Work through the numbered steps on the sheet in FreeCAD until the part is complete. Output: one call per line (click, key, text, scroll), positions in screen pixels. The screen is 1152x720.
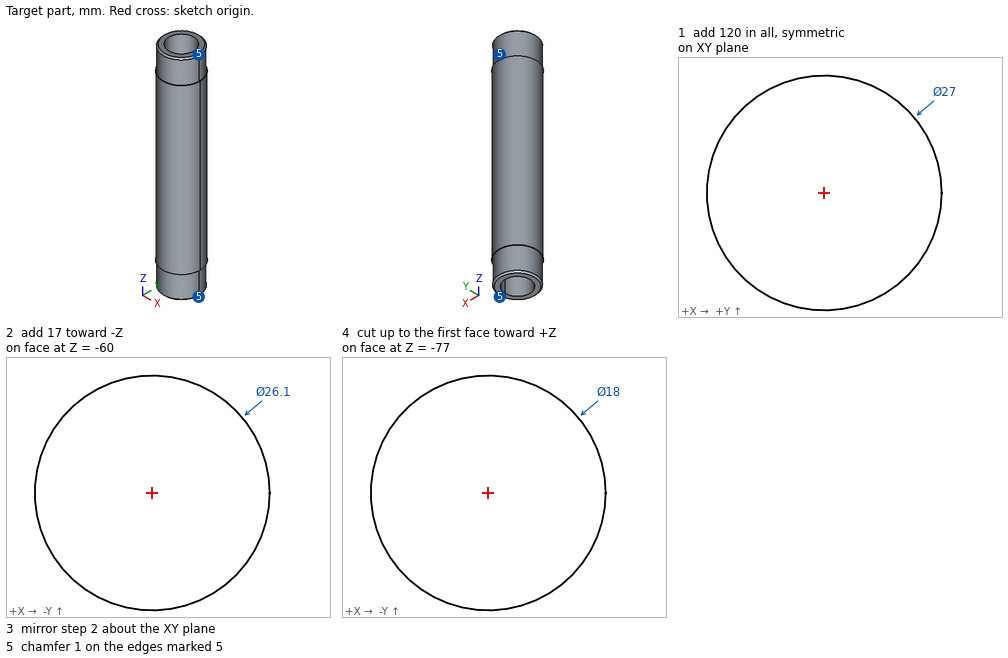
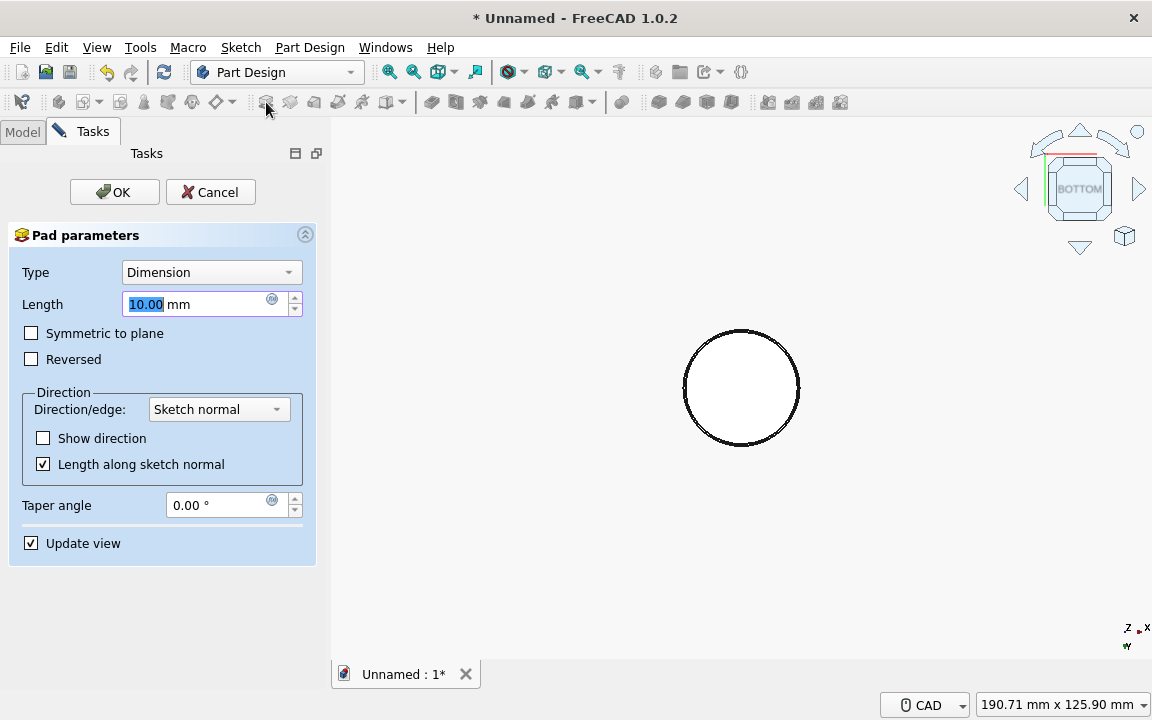
text(17)
key(Tab)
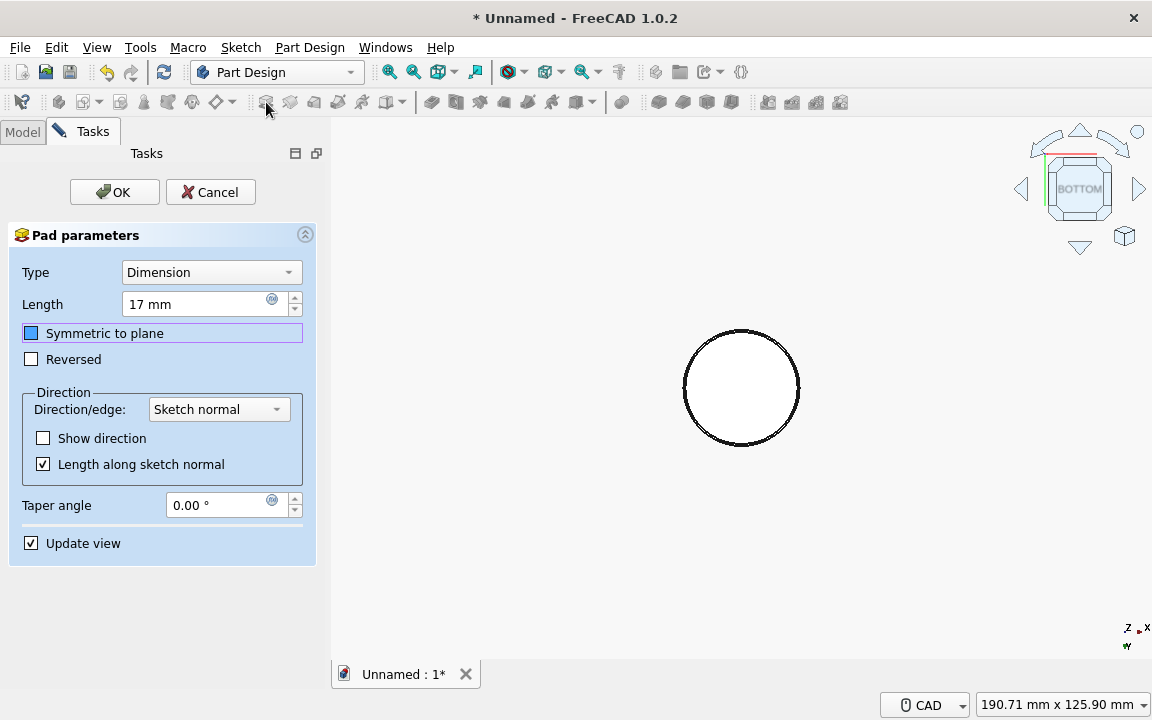
click(115, 192)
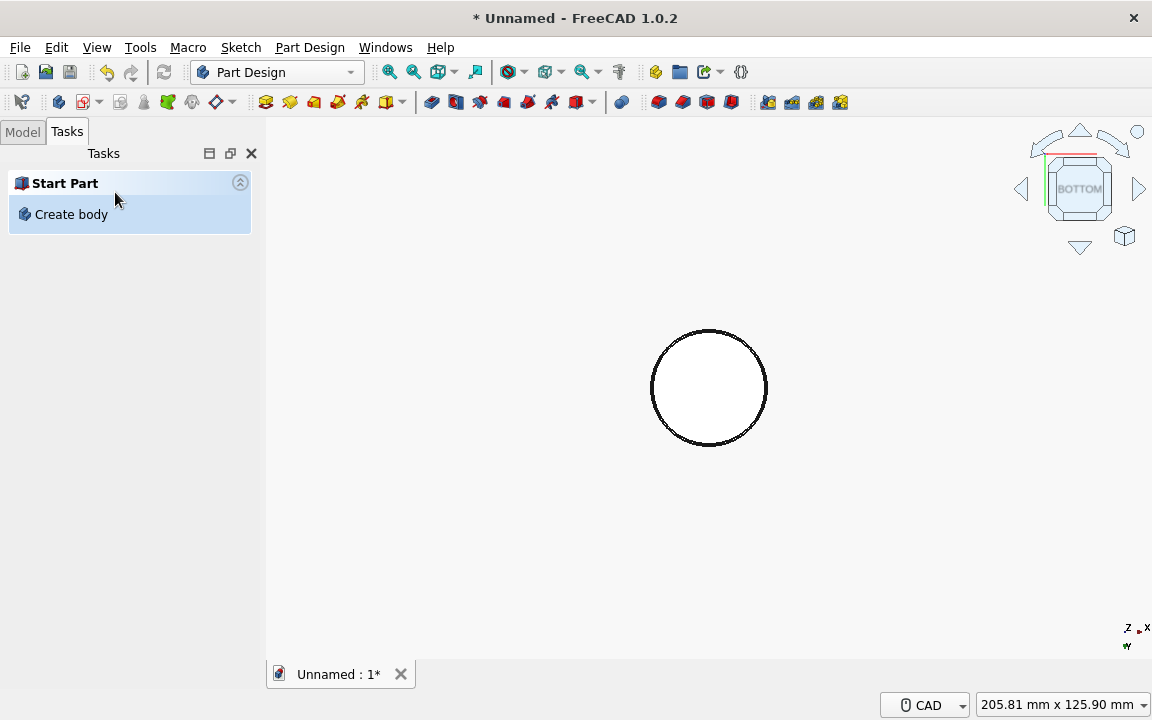
key(v)
key(f)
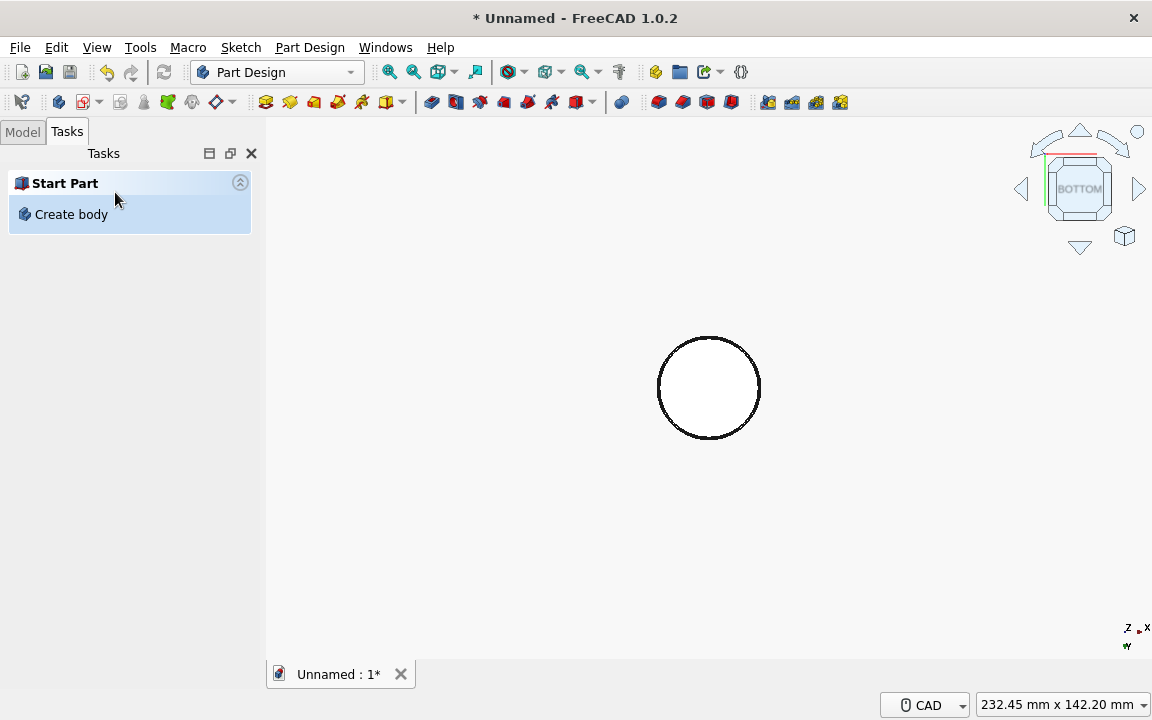
click(23, 131)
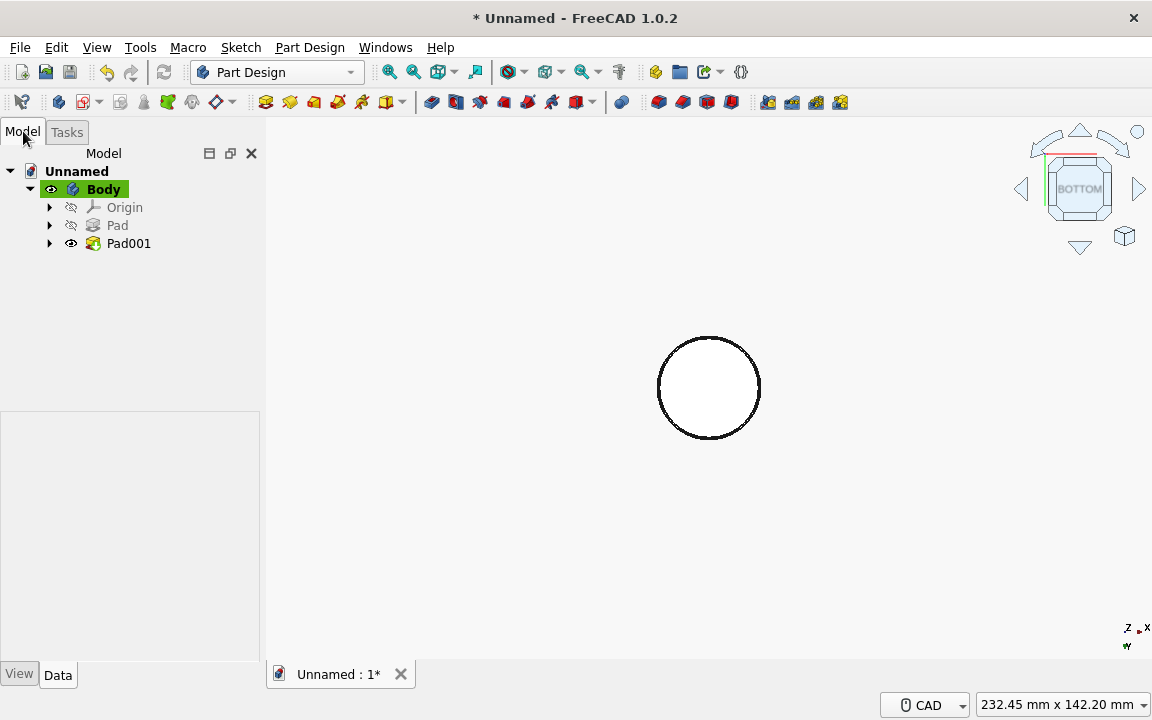
click(116, 243)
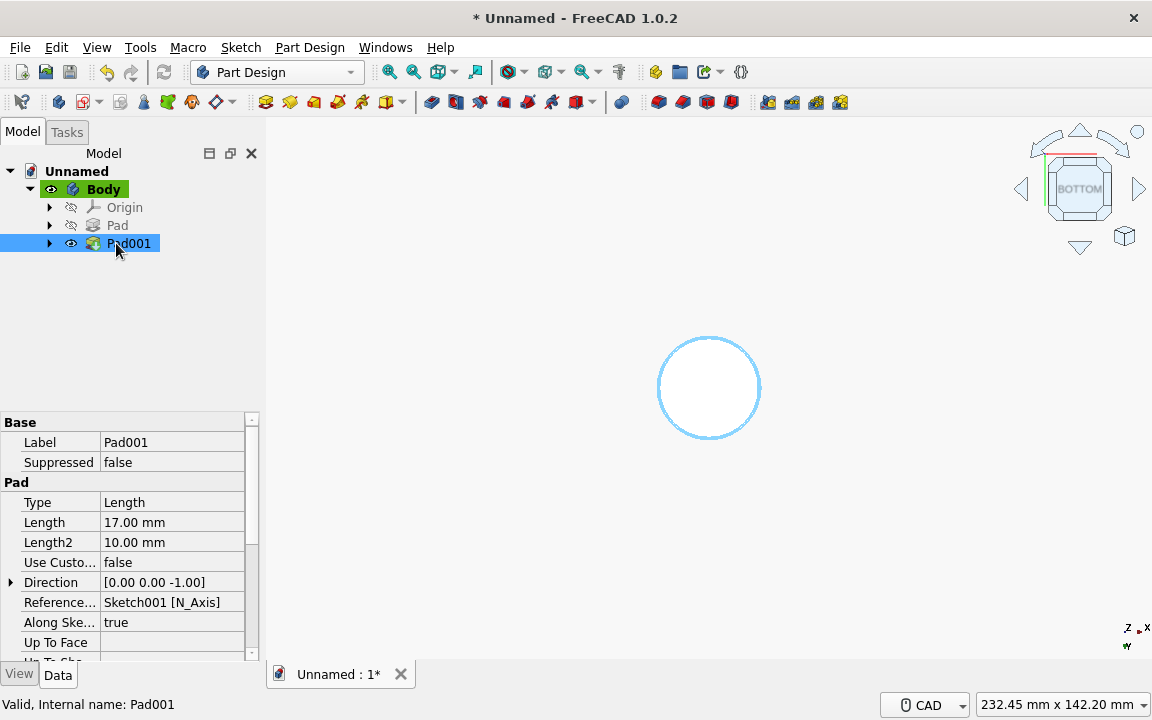
click(768, 102)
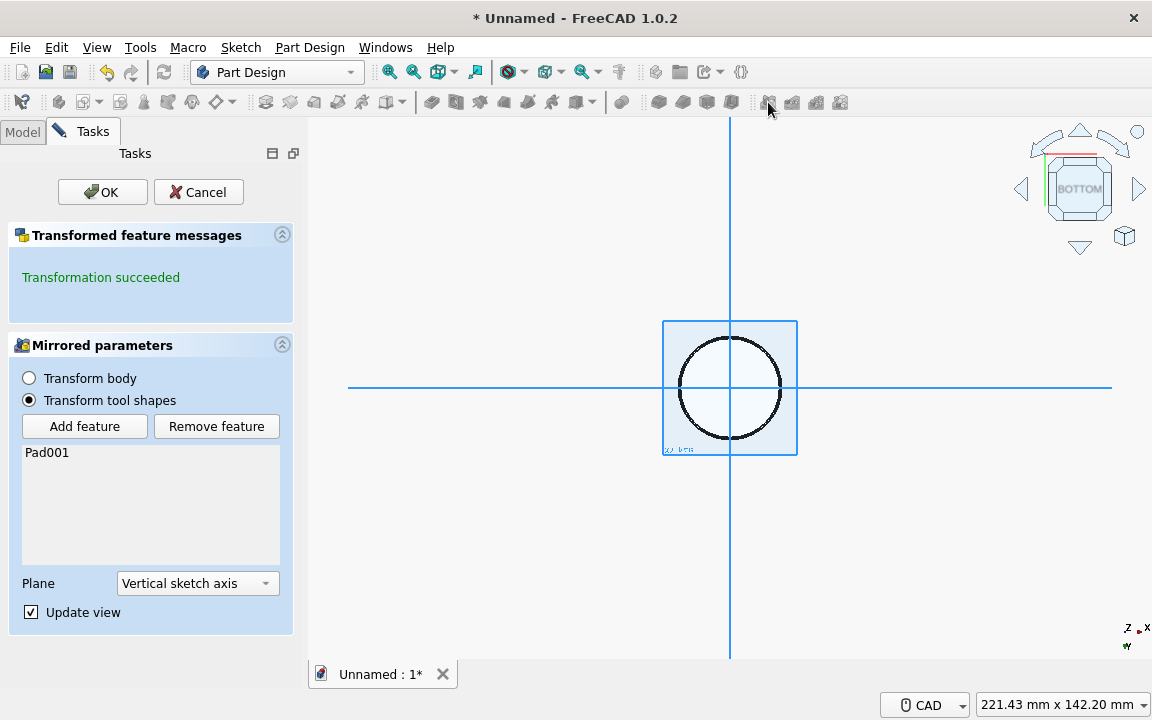
click(198, 584)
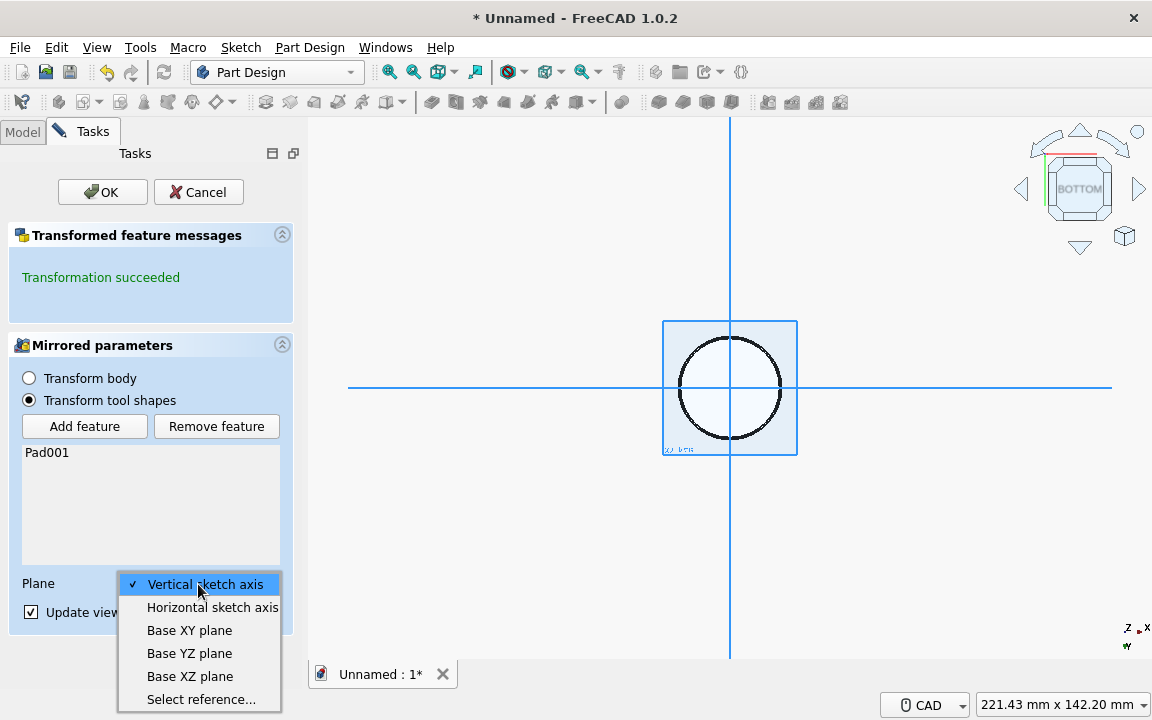
click(198, 630)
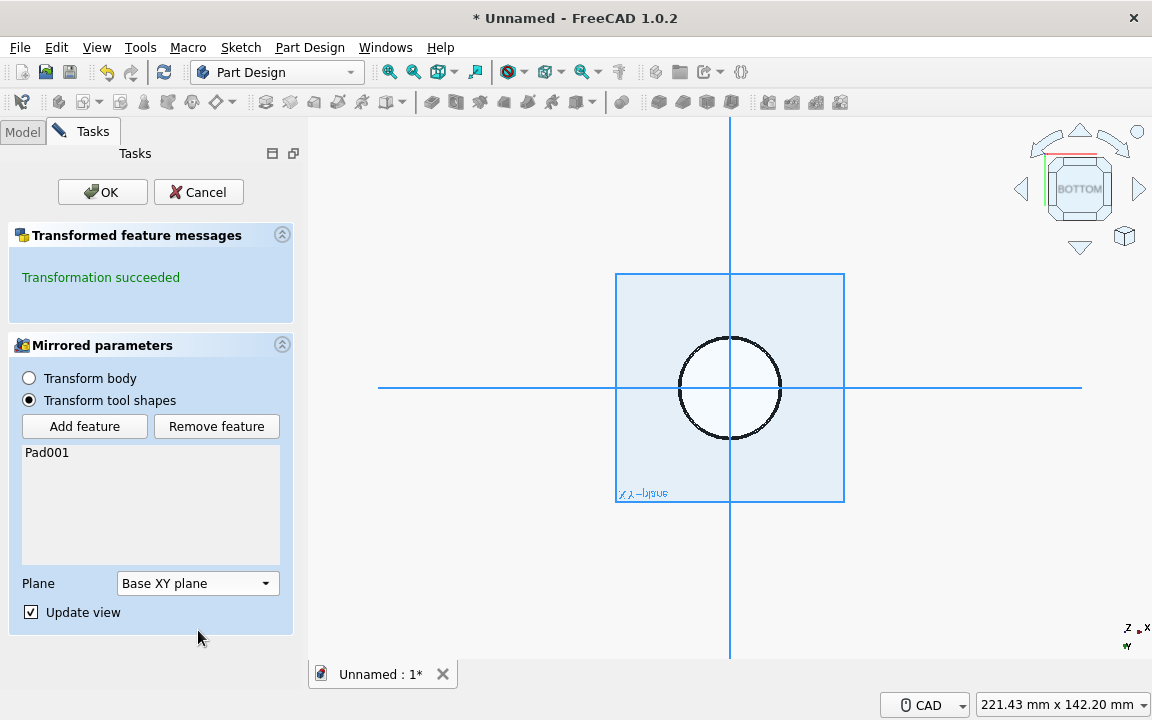
click(103, 192)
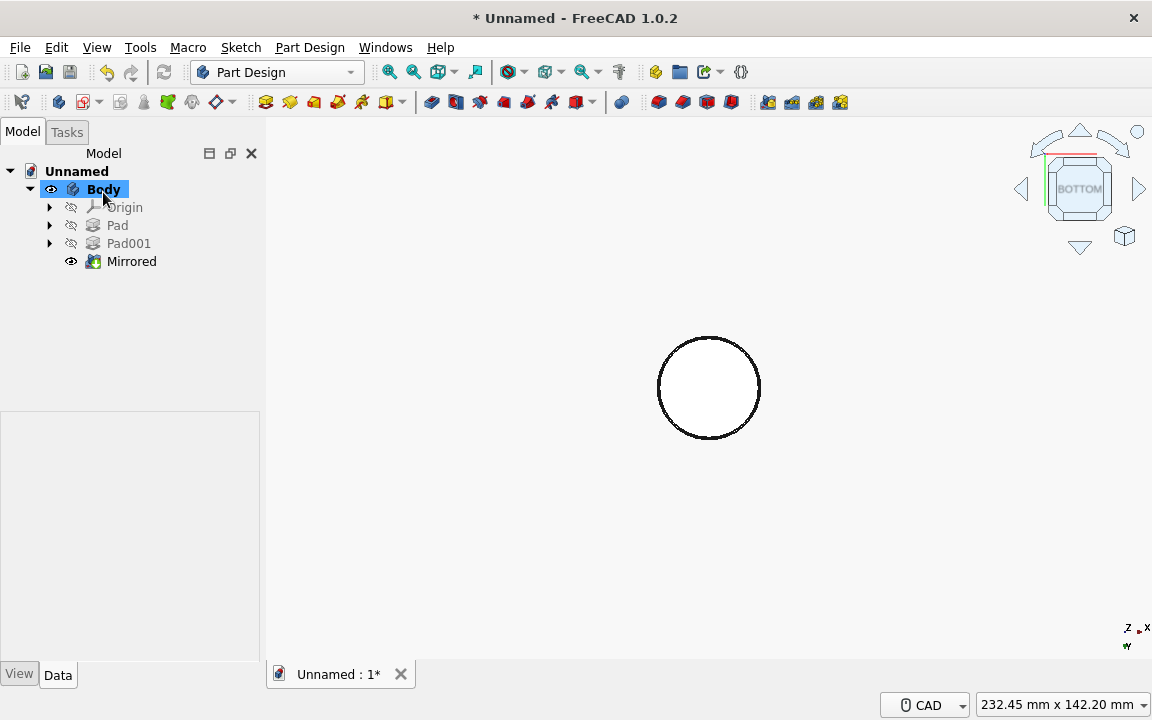
key(v)
key(f)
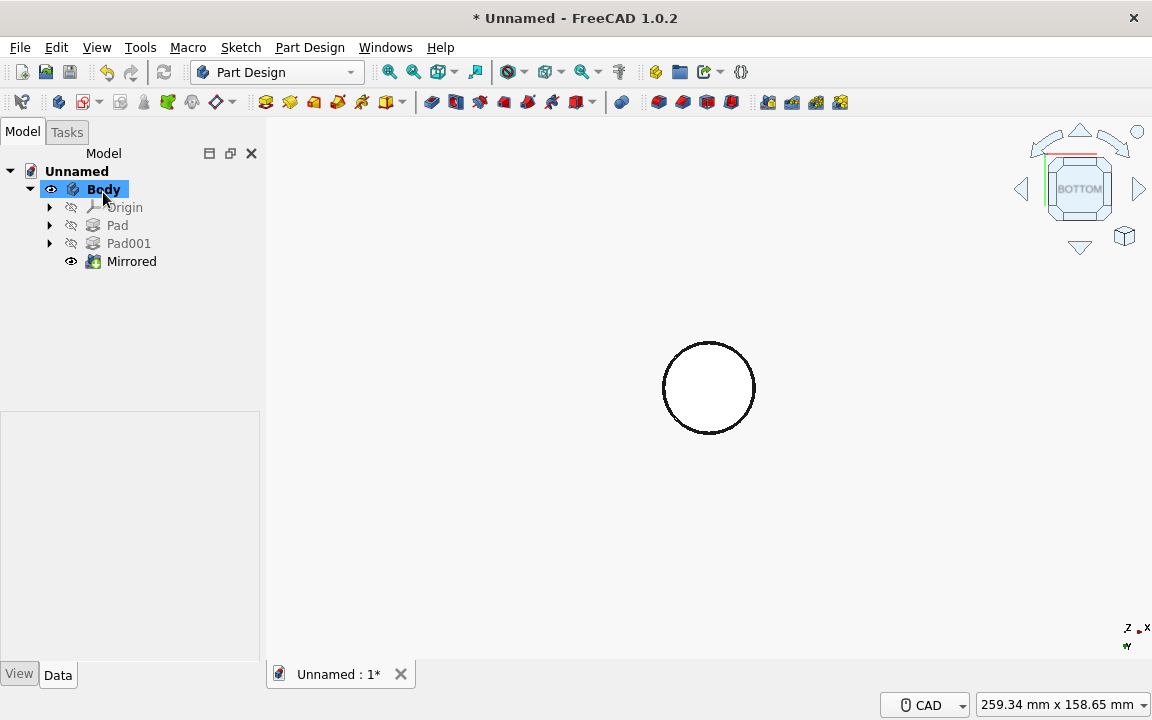
click(709, 387)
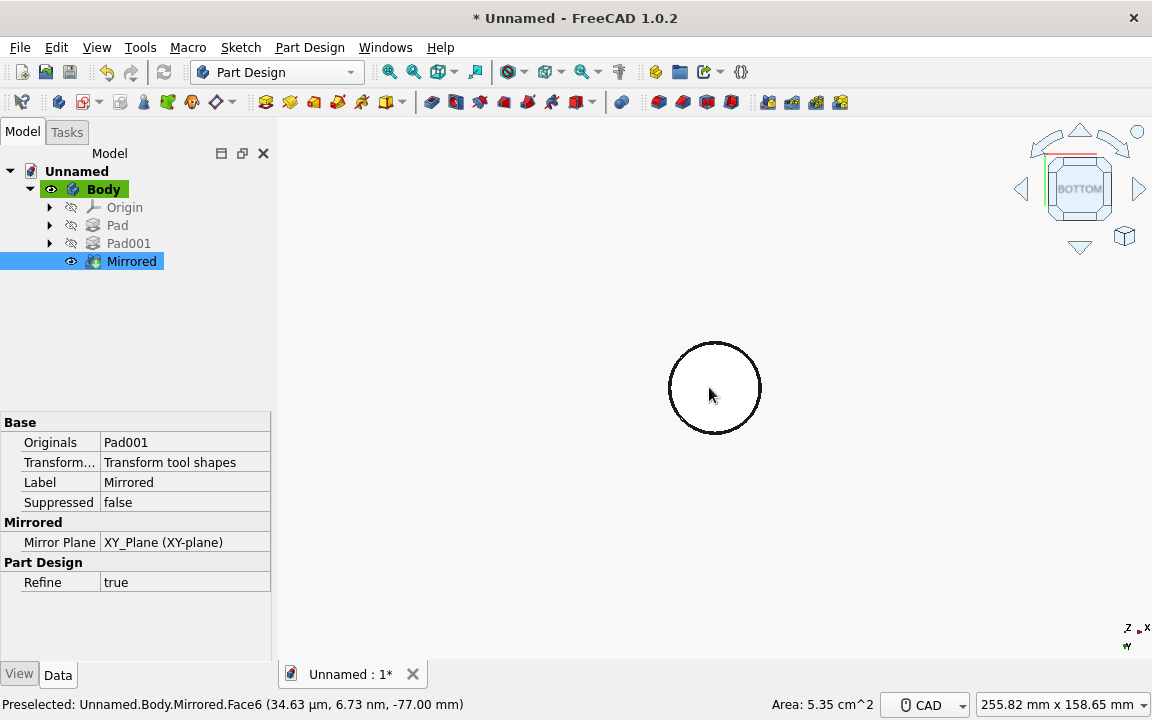
click(84, 102)